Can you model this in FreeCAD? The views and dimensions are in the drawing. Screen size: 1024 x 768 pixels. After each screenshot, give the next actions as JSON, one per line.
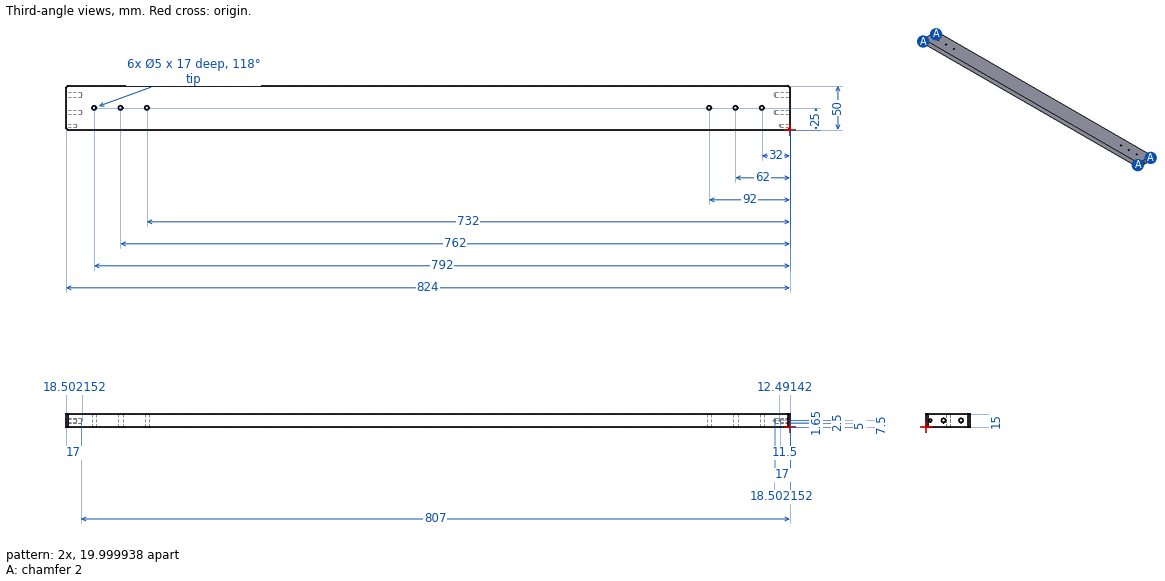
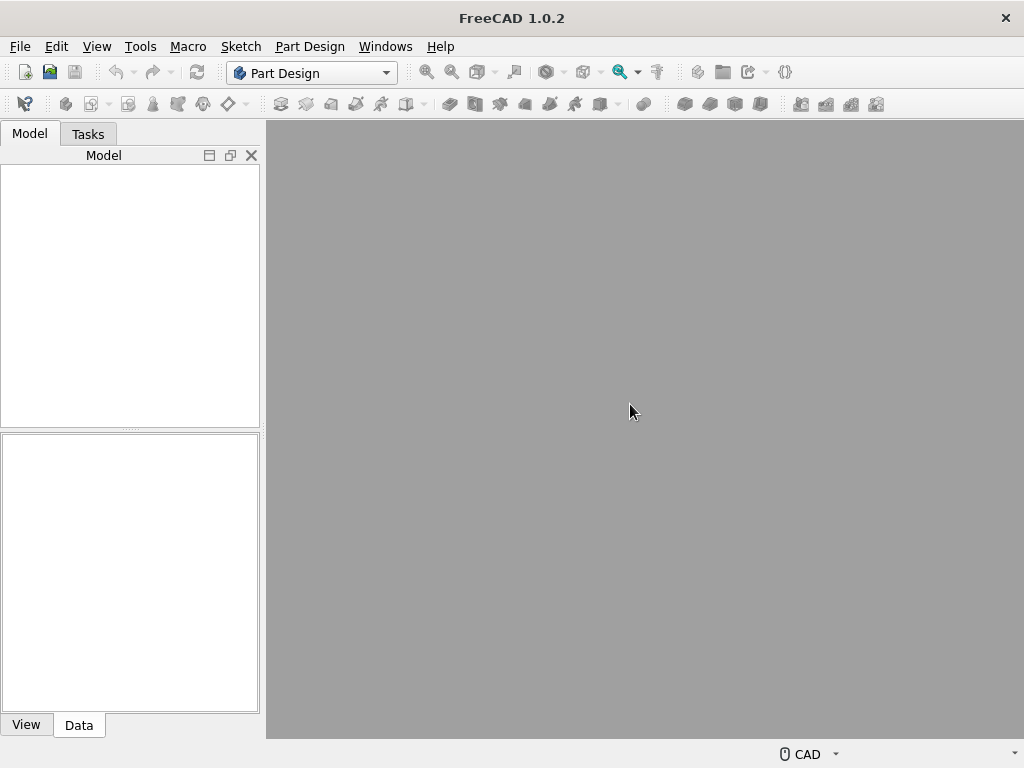
{"action": "left_click", "coordinate": [25, 72]}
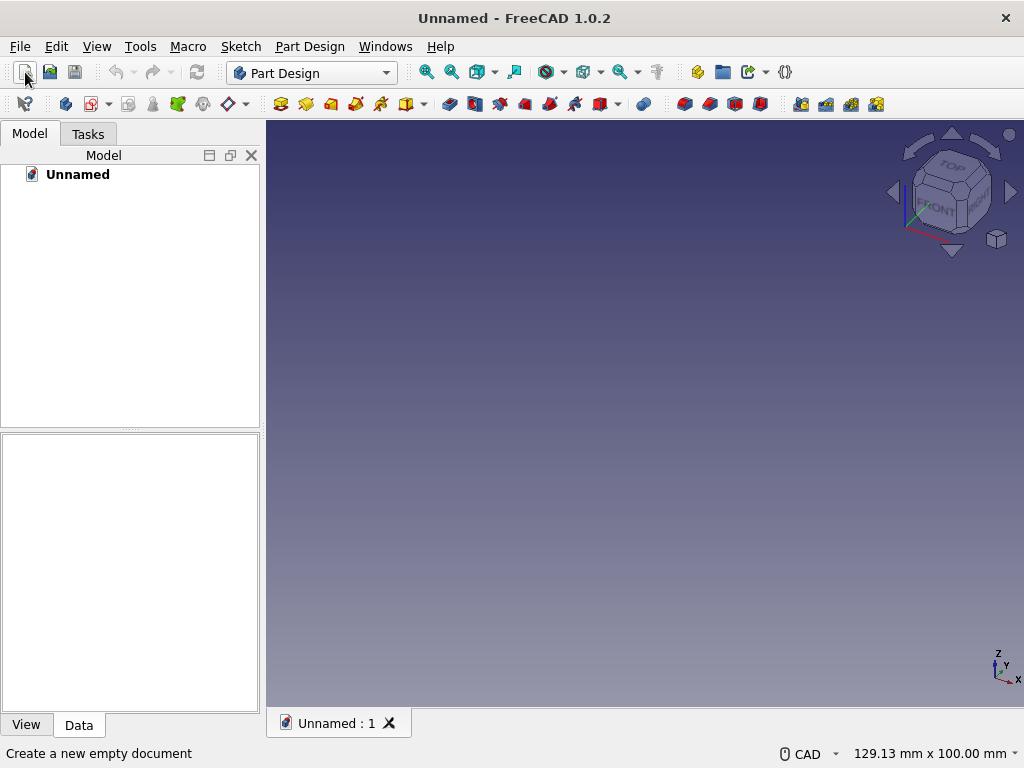
{"action": "left_click", "coordinate": [90, 104]}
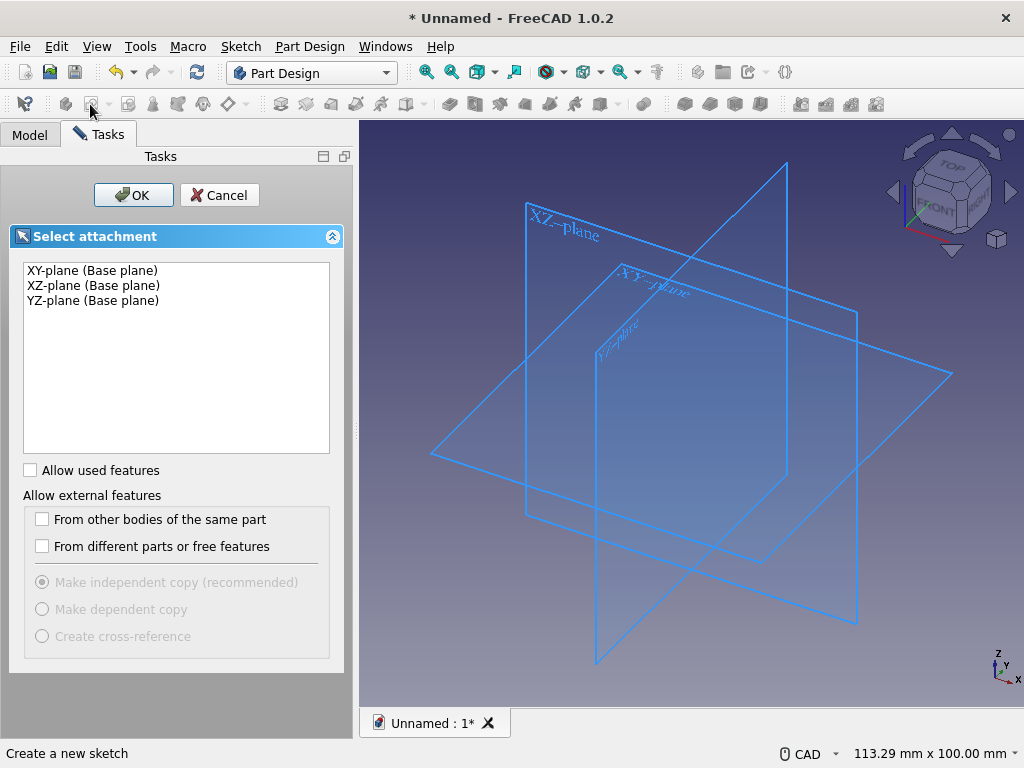
{"action": "left_click", "coordinate": [84, 270]}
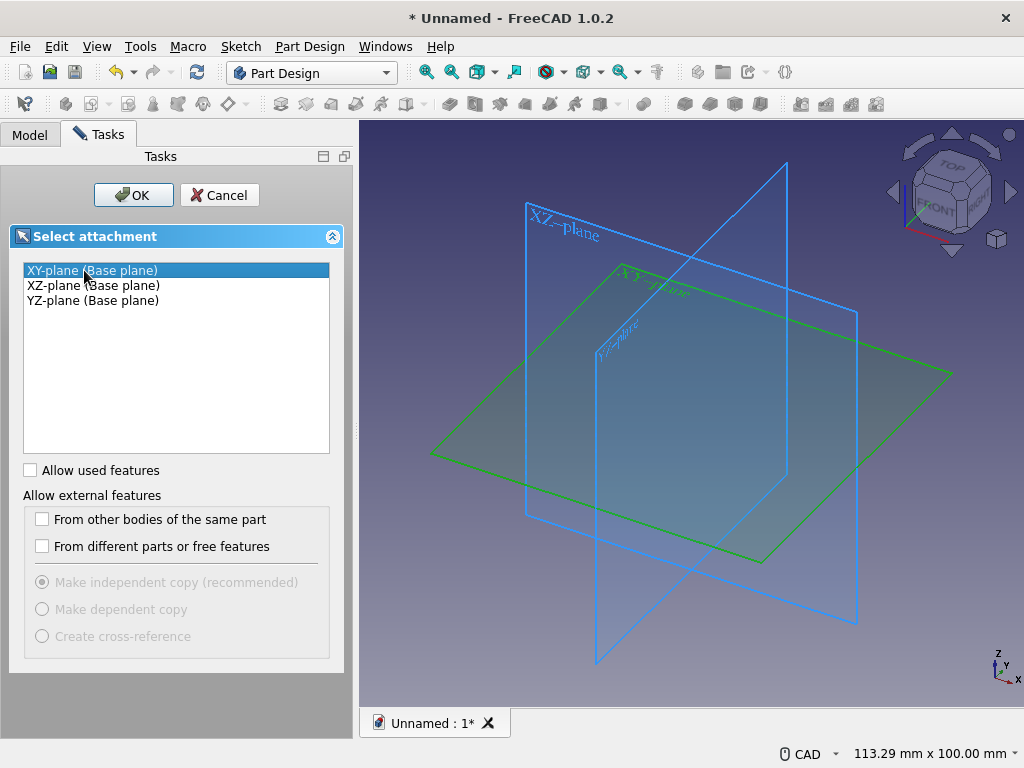
{"action": "left_click", "coordinate": [134, 195]}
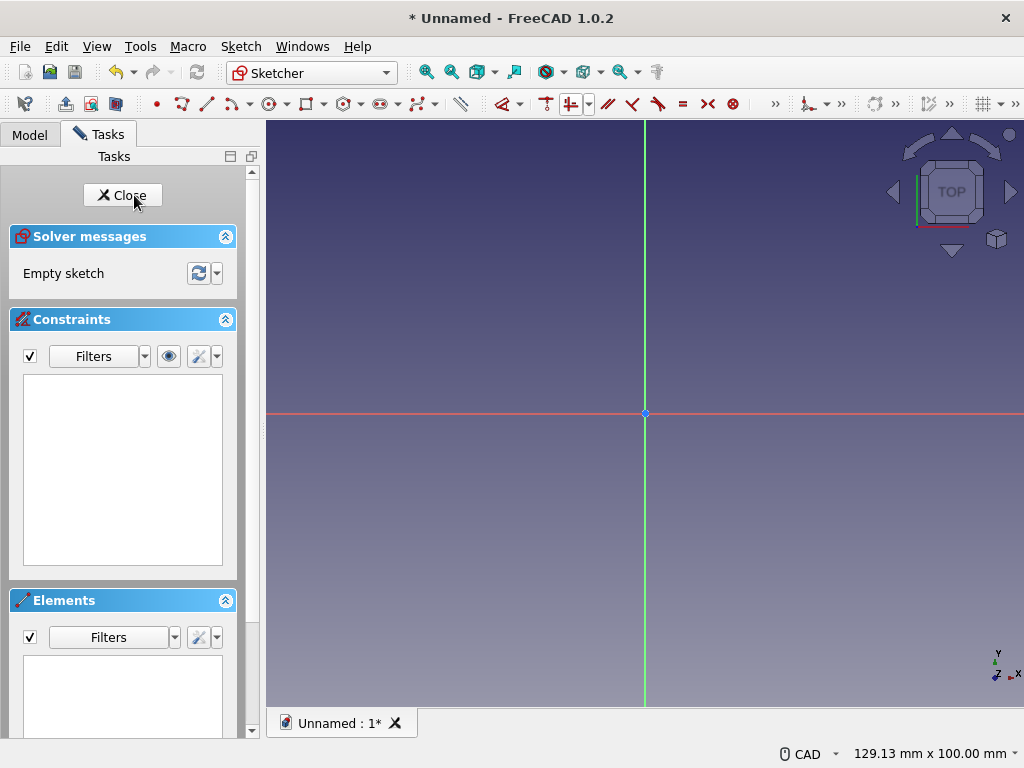
{"action": "scroll", "coordinate": [811, 428], "scroll_direction": "down", "scroll_amount": 12}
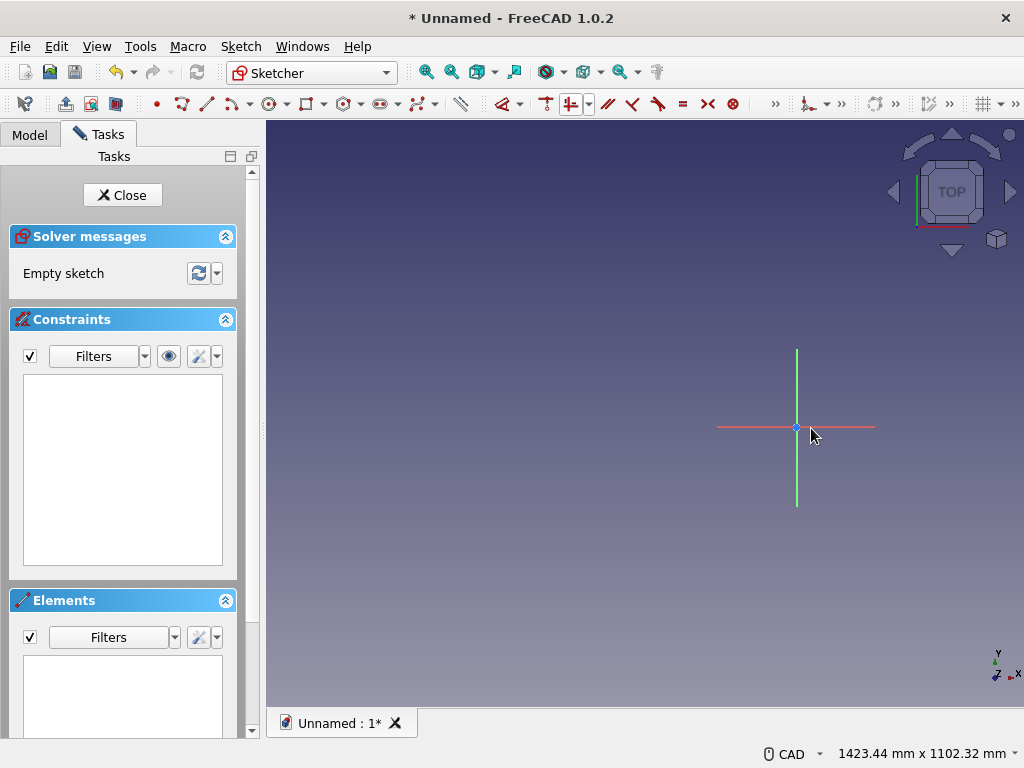
{"action": "left_click", "coordinate": [306, 104]}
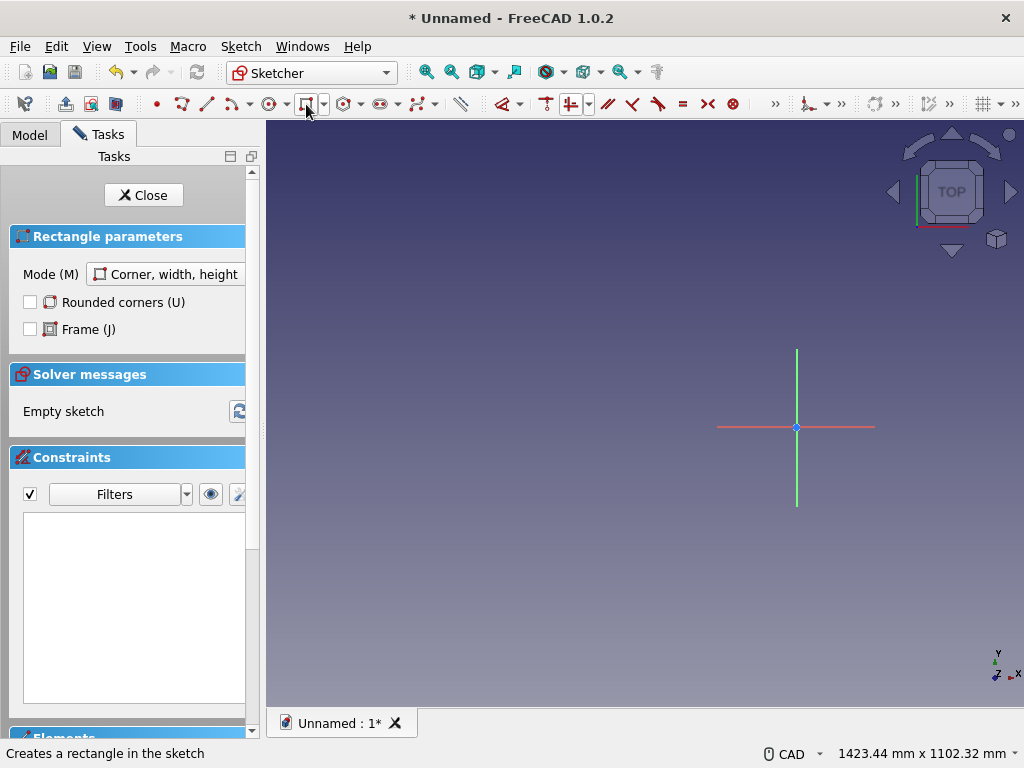
{"action": "left_click", "coordinate": [797, 427]}
{"action": "mouse_move", "coordinate": [358, 401]}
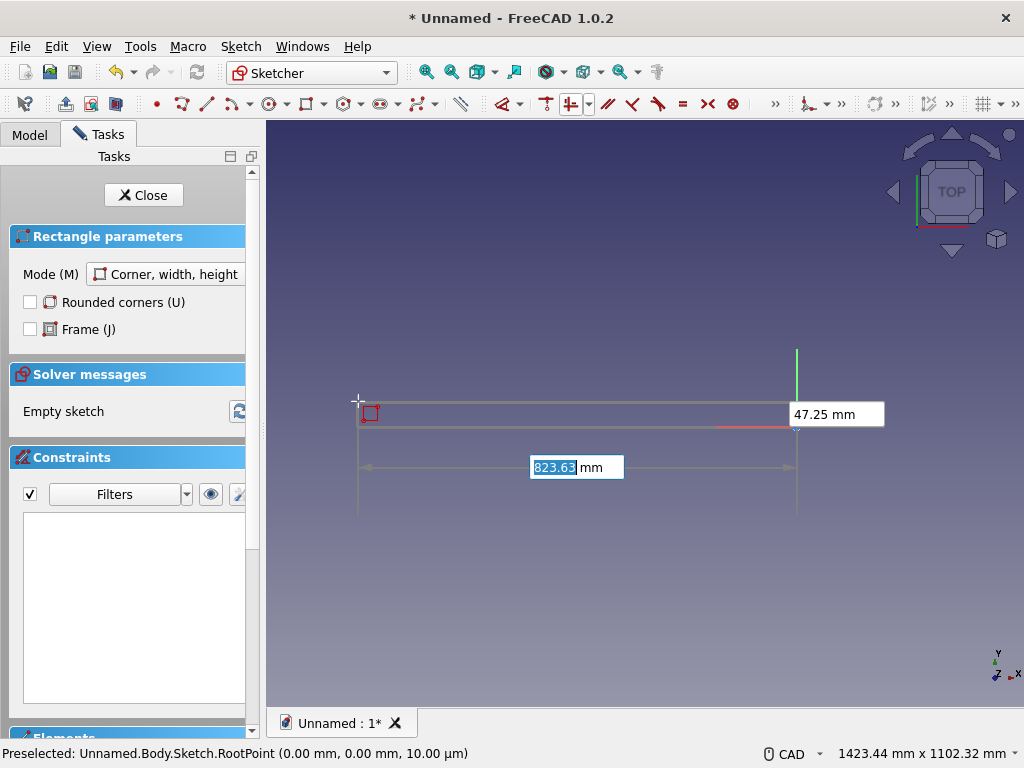
{"action": "type", "text": "824"}
{"action": "key", "text": "Tab"}
{"action": "type", "text": "50"}
{"action": "key", "text": "Return"}
{"action": "key", "text": "Escape"}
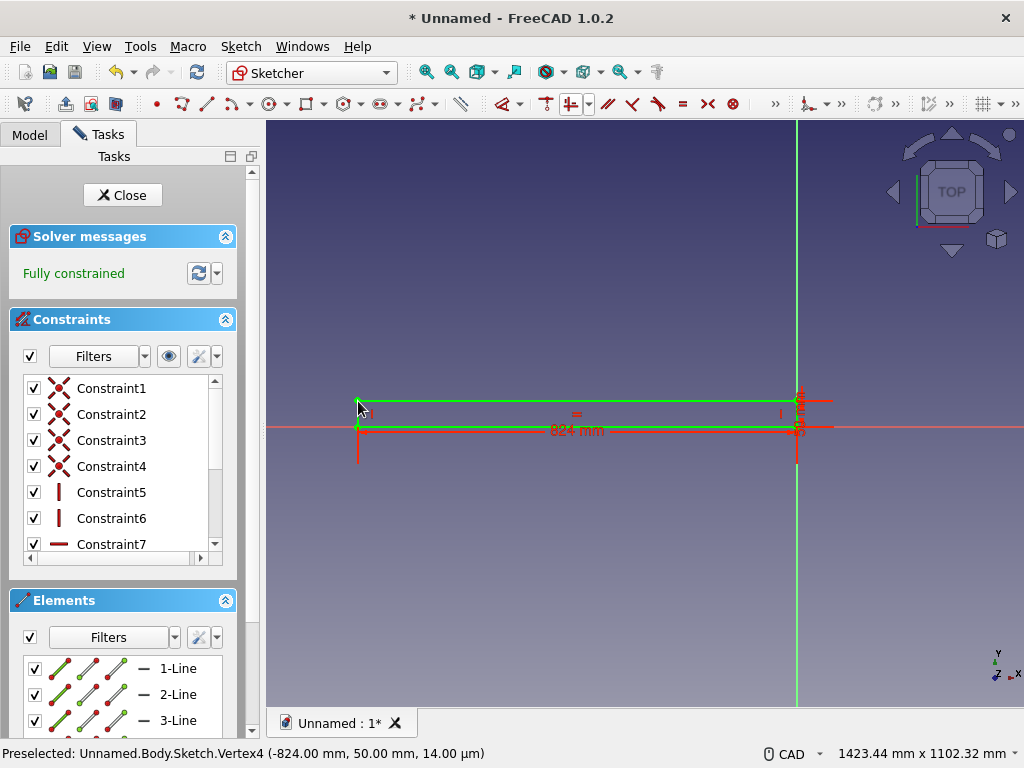
{"action": "left_click", "coordinate": [123, 195]}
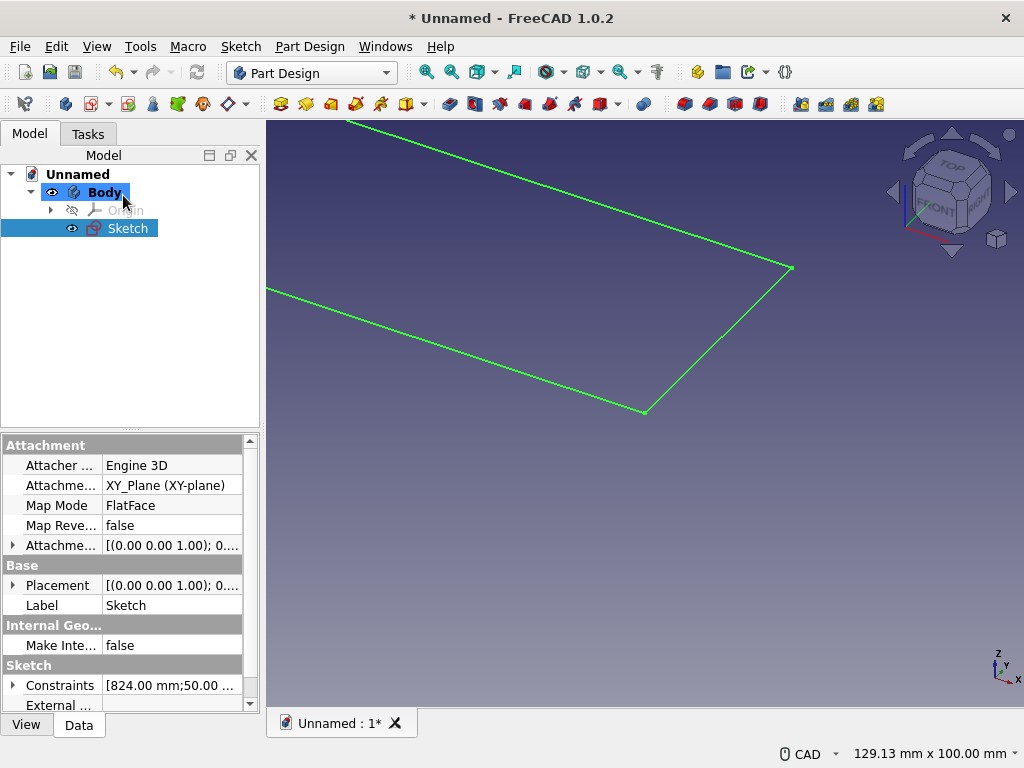
{"action": "left_click", "coordinate": [281, 104]}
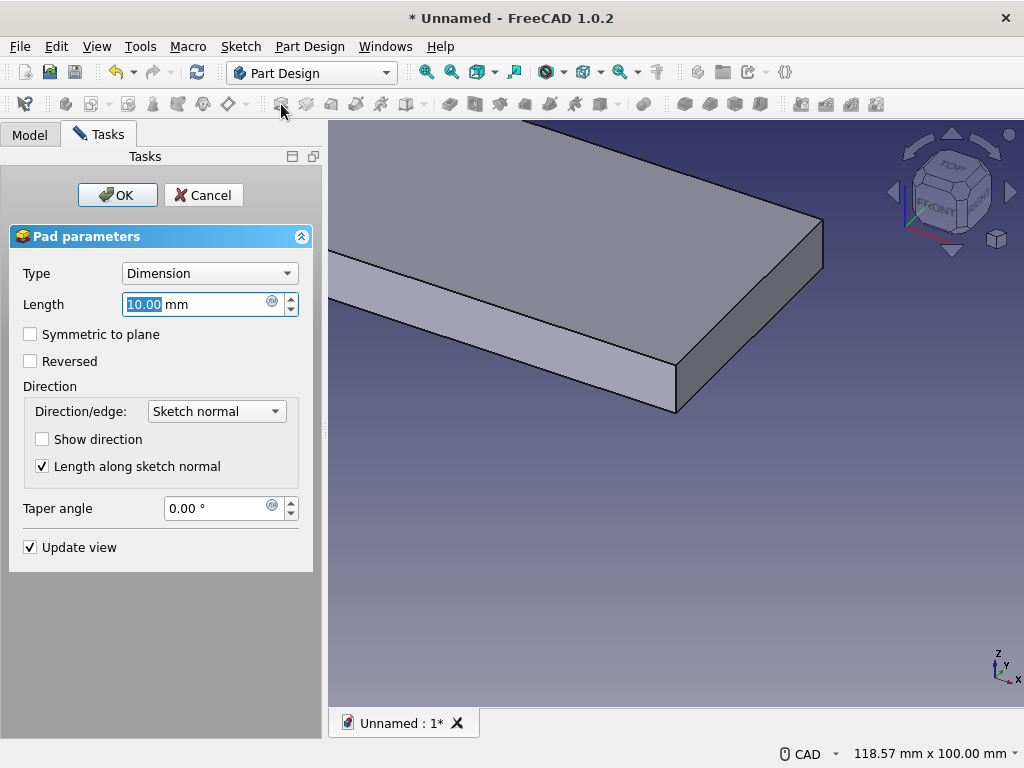
{"action": "type", "text": "15"}
{"action": "key", "text": "Tab"}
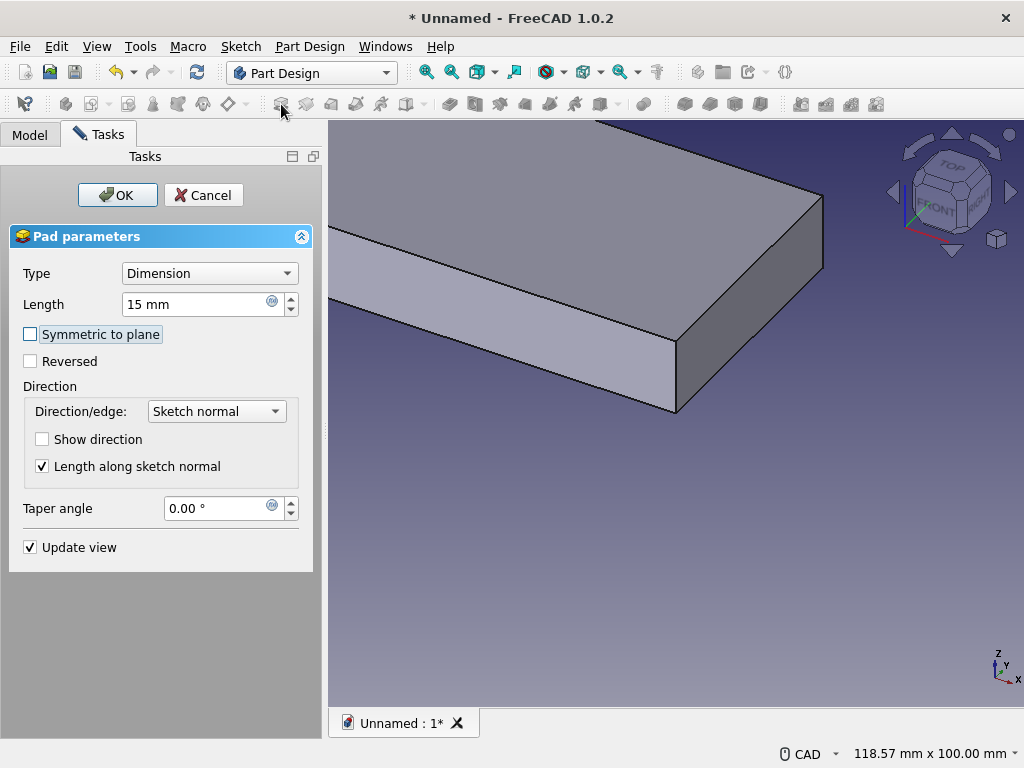
{"action": "left_click", "coordinate": [118, 195]}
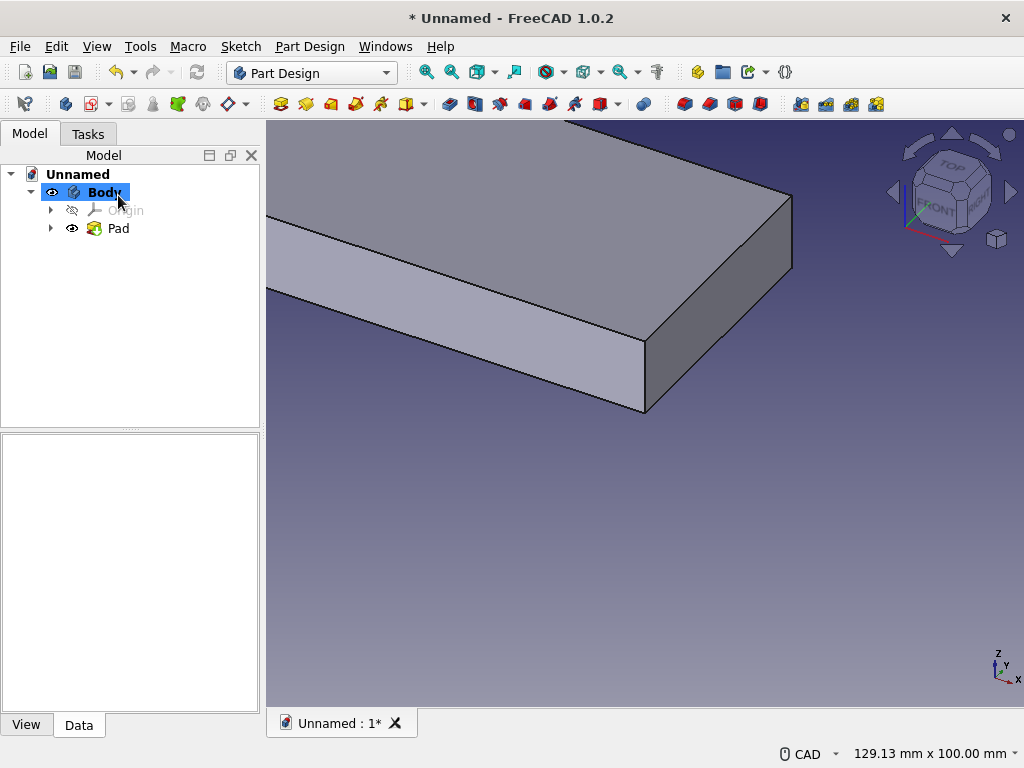
{"action": "left_click", "coordinate": [427, 72]}